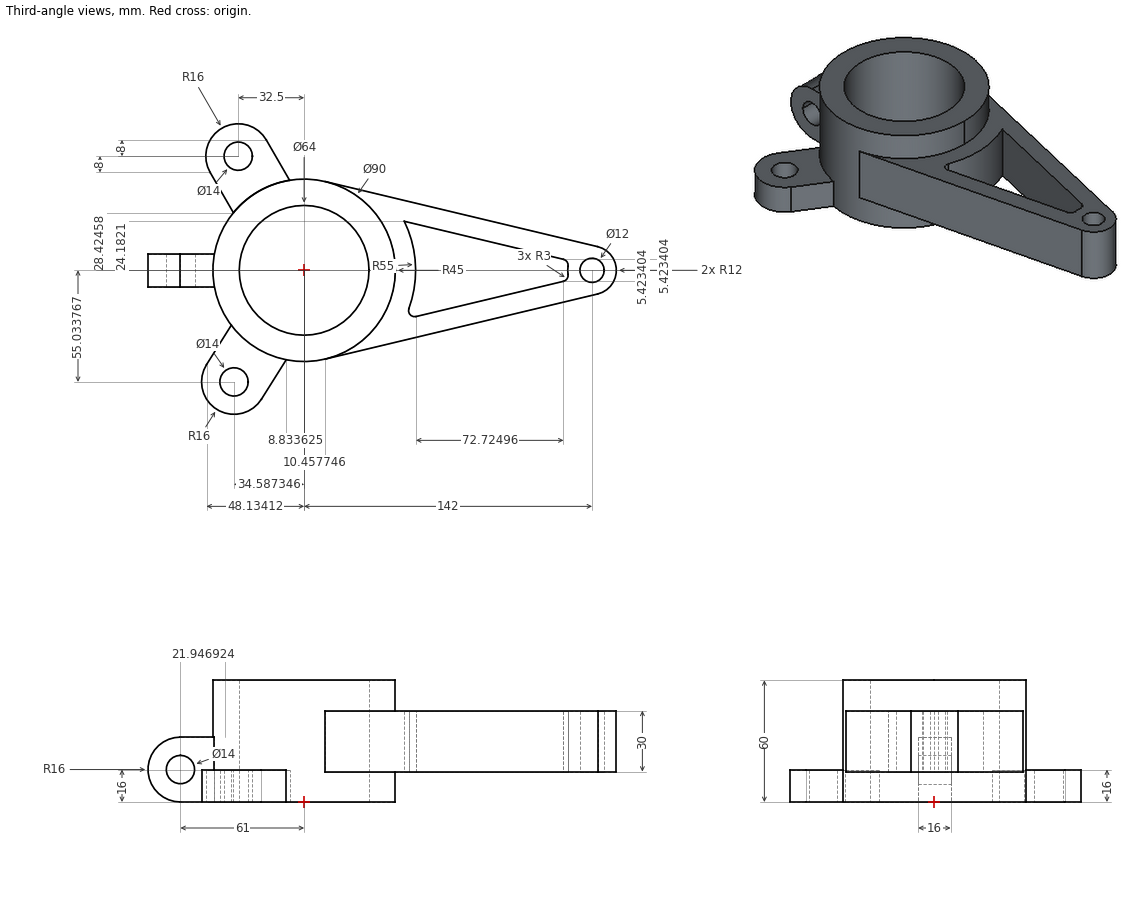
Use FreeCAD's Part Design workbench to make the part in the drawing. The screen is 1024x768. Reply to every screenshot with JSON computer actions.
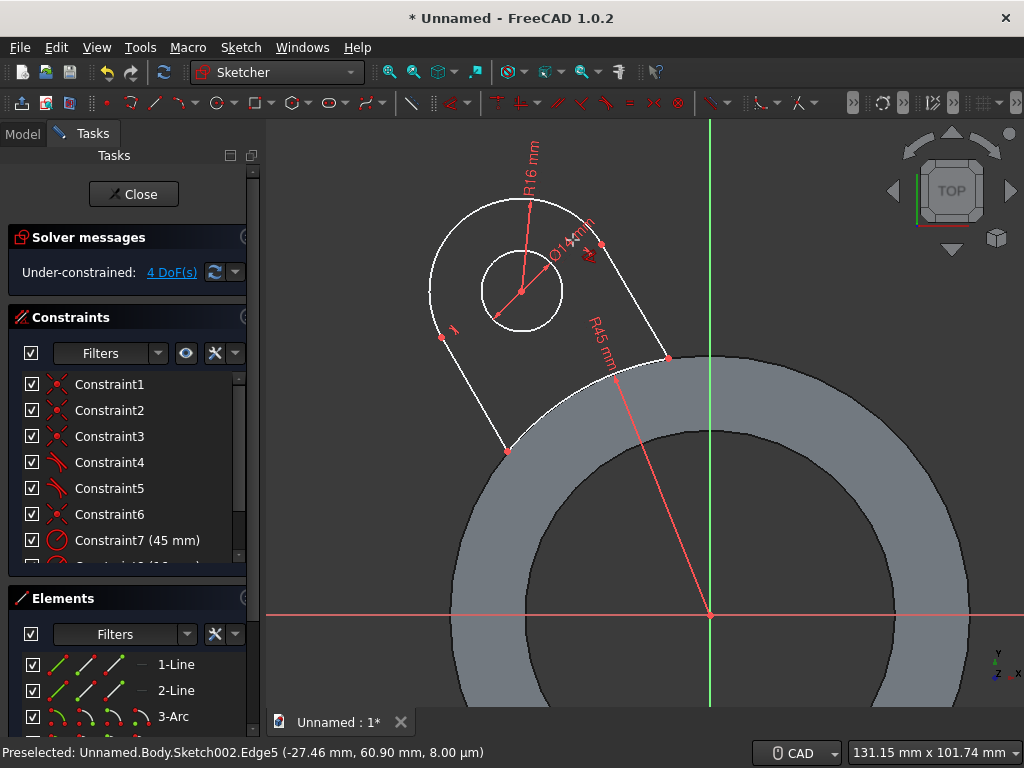
{"action": "left_click", "coordinate": [602, 244]}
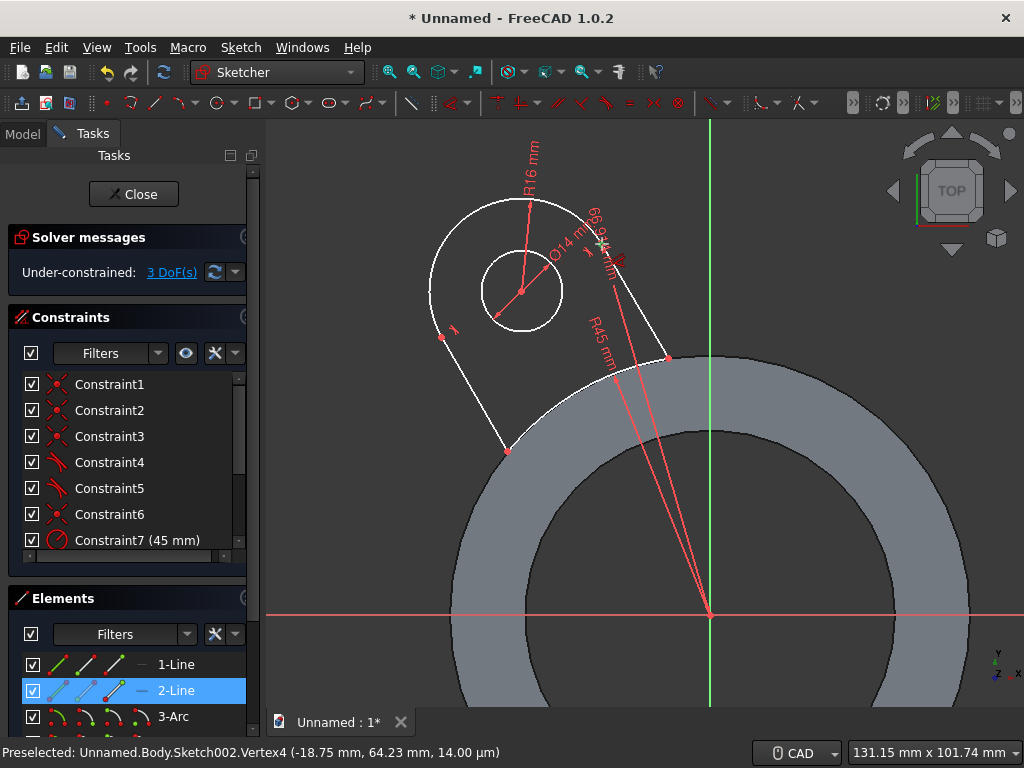
{"action": "left_click", "coordinate": [522, 291]}
{"action": "left_click", "coordinate": [636, 268]}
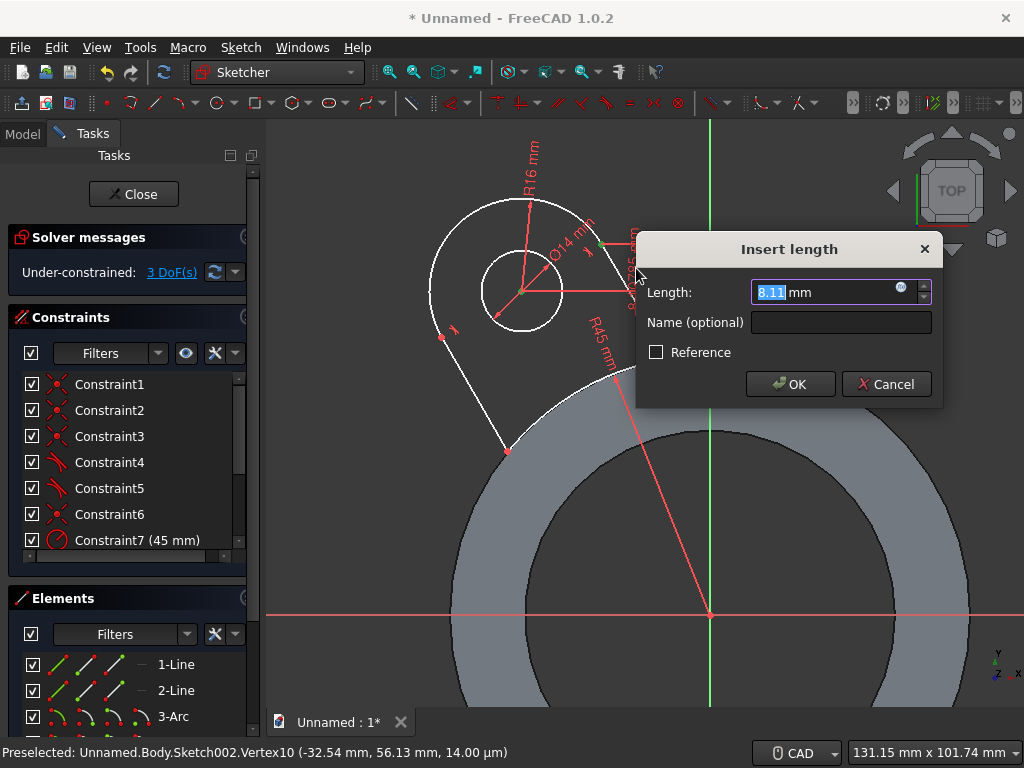
{"action": "type", "text": "8"}
{"action": "key", "text": "Return"}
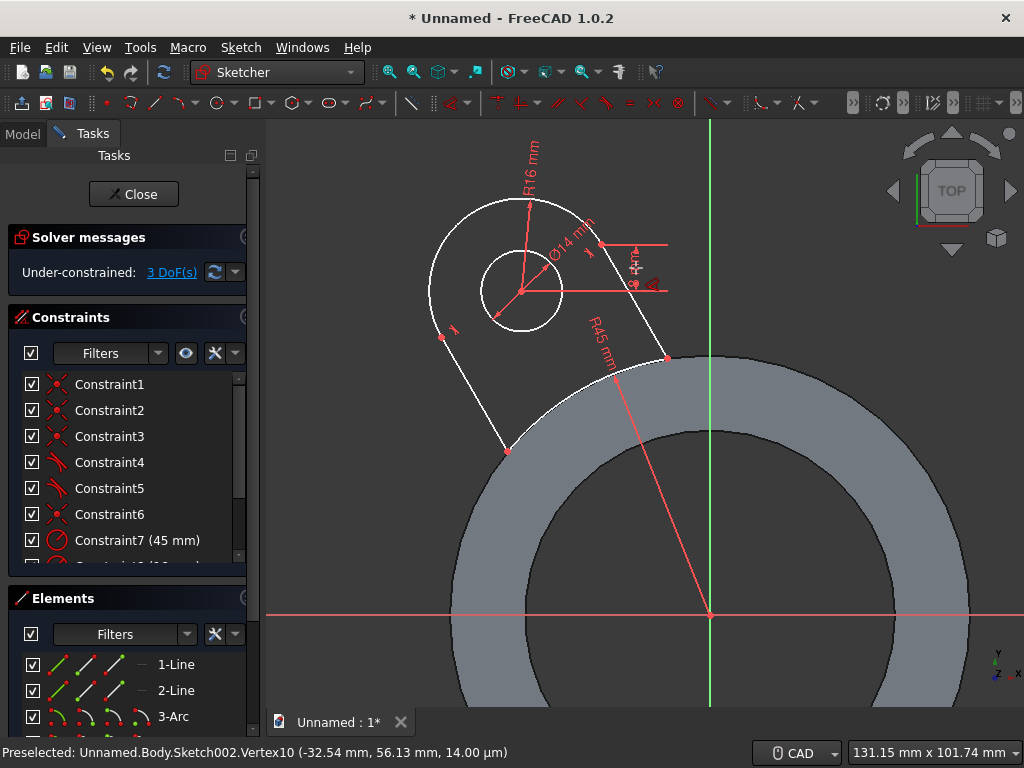
{"action": "left_click", "coordinate": [442, 337]}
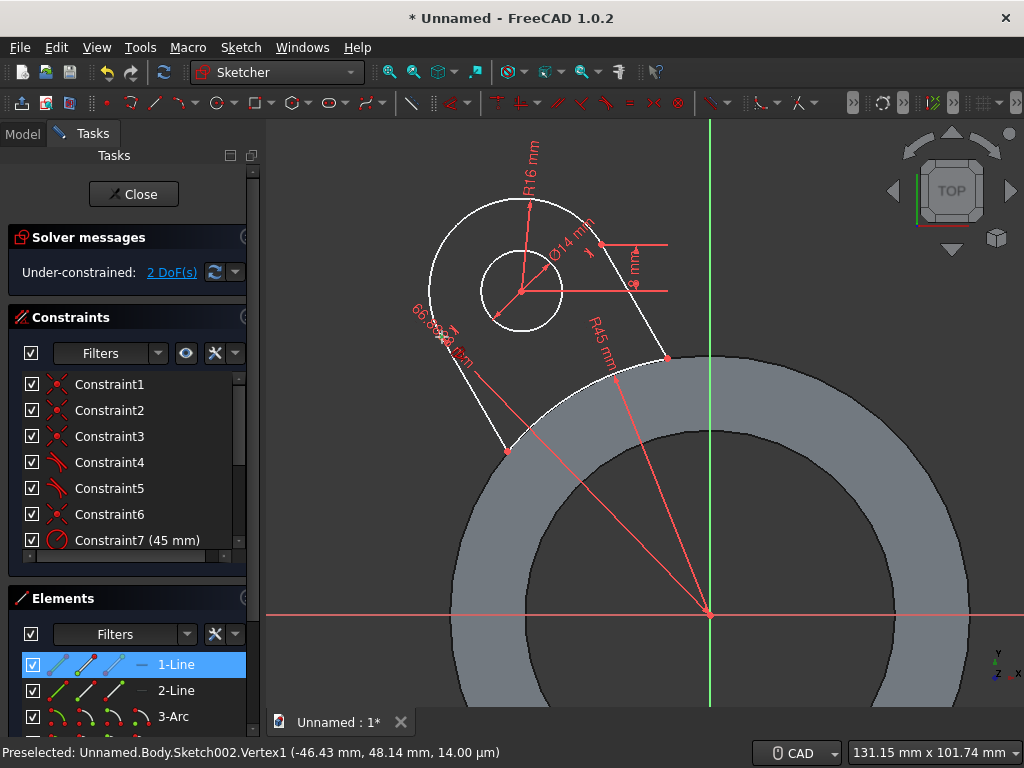
{"action": "left_click", "coordinate": [522, 291]}
{"action": "left_click", "coordinate": [408, 314]}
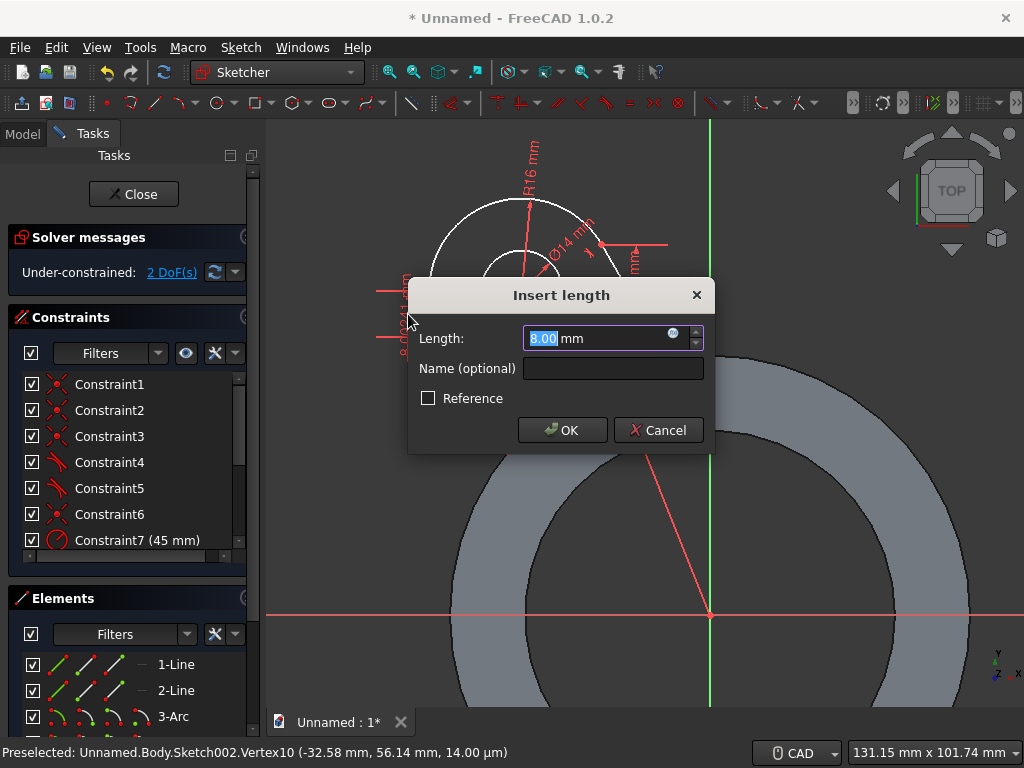
{"action": "type", "text": "8"}
{"action": "key", "text": "Return"}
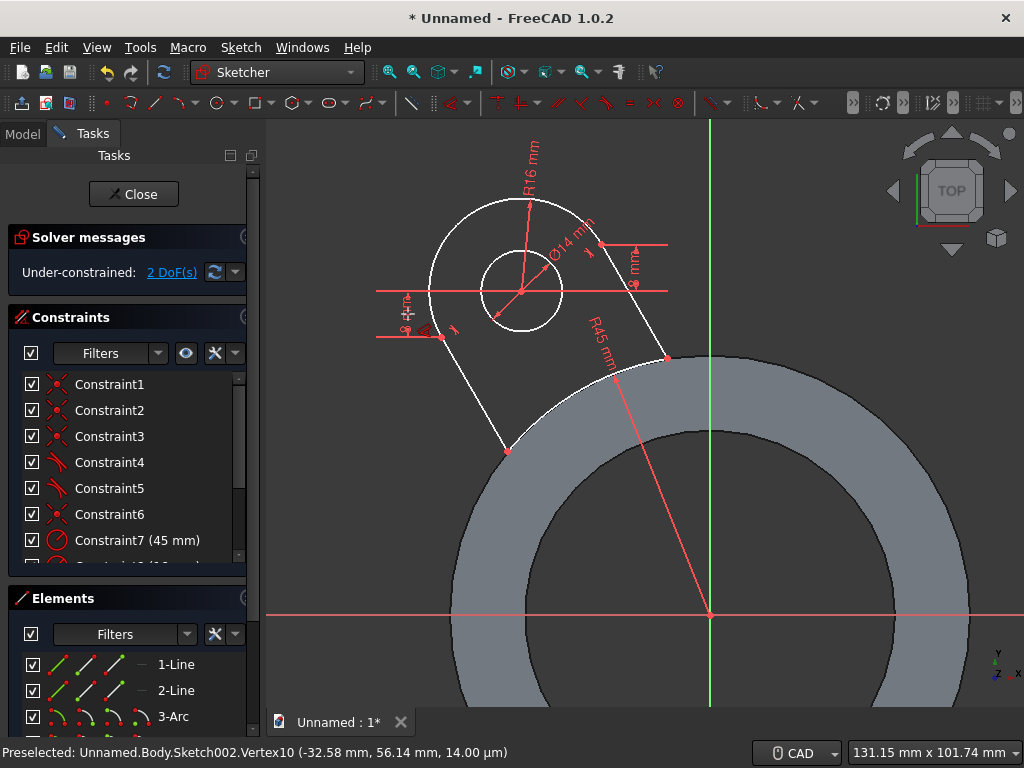
{"action": "left_click", "coordinate": [522, 291]}
{"action": "left_click", "coordinate": [616, 649]}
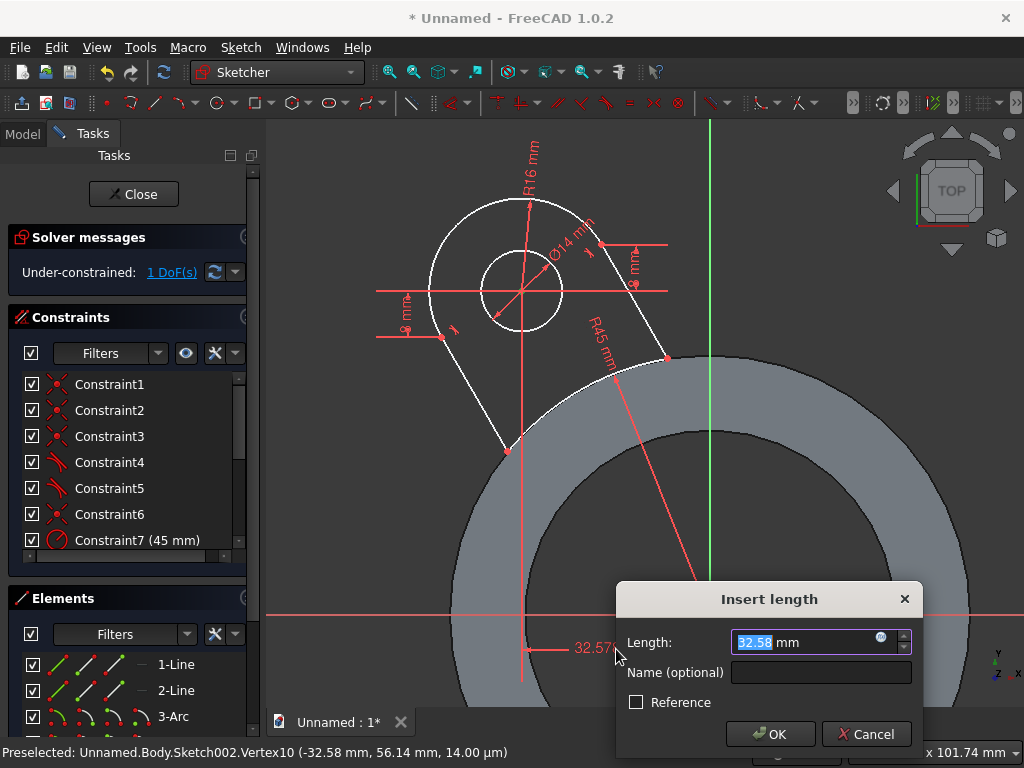
{"action": "type", "text": "32.5"}
{"action": "key", "text": "Return"}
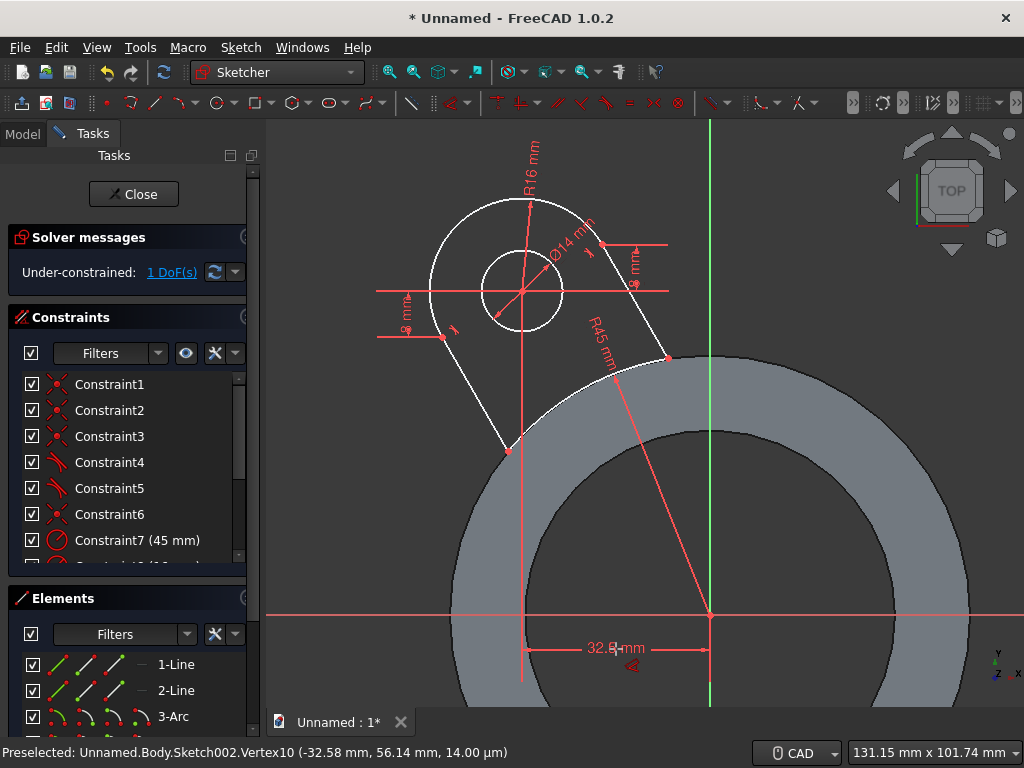
{"action": "left_click", "coordinate": [508, 452]}
{"action": "left_click", "coordinate": [744, 534]}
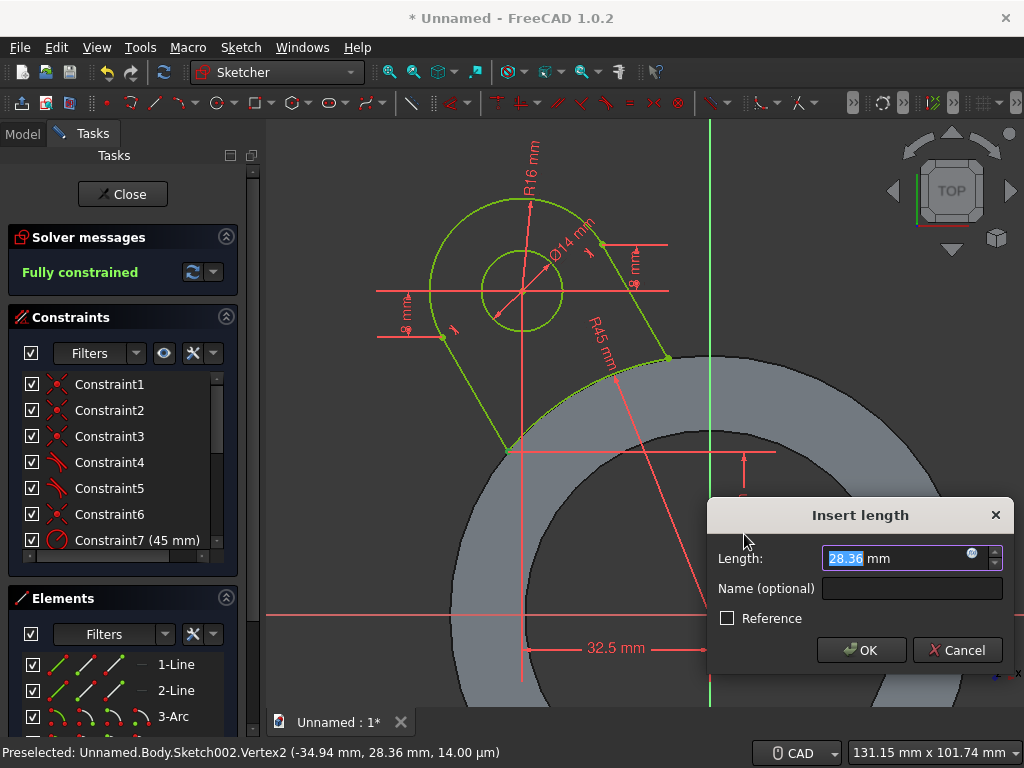
{"action": "type", "text": "28.42458"}
{"action": "key", "text": "Return"}
{"action": "key", "text": "Escape"}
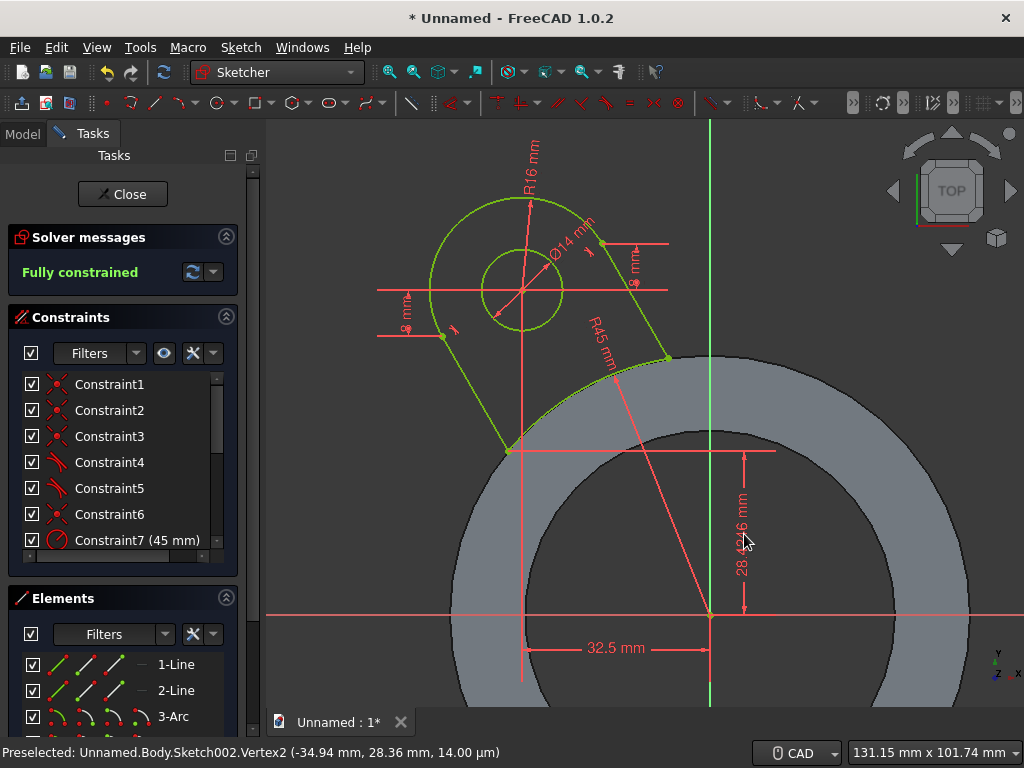
{"action": "left_click", "coordinate": [123, 194]}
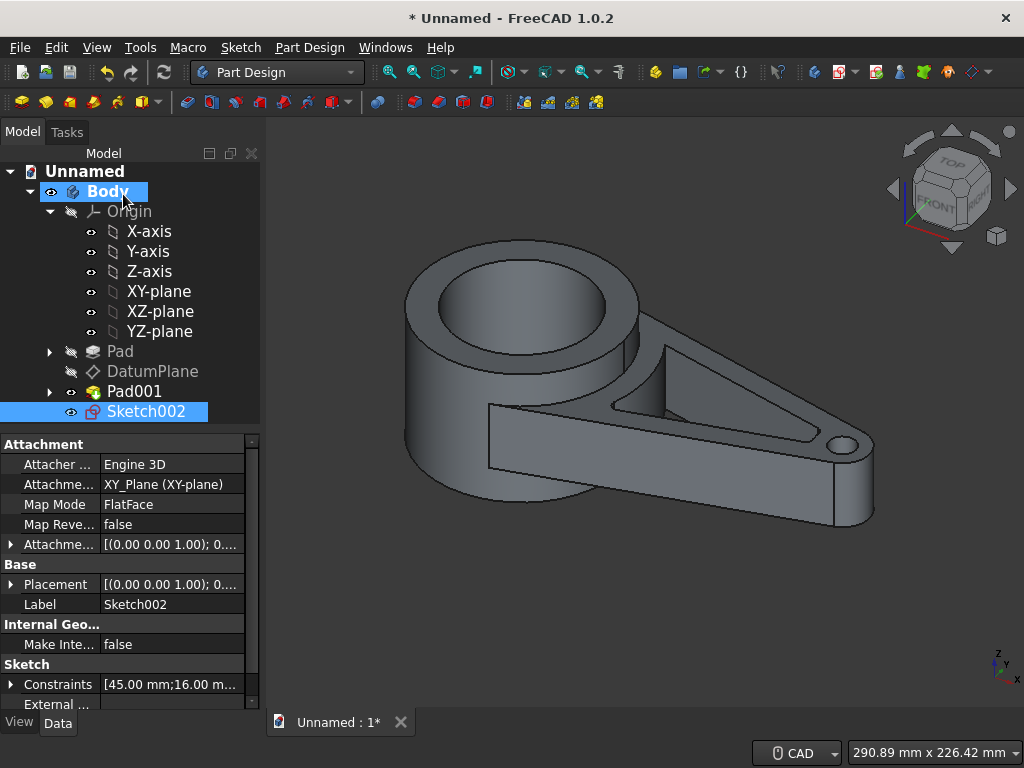
{"action": "left_click", "coordinate": [22, 102]}